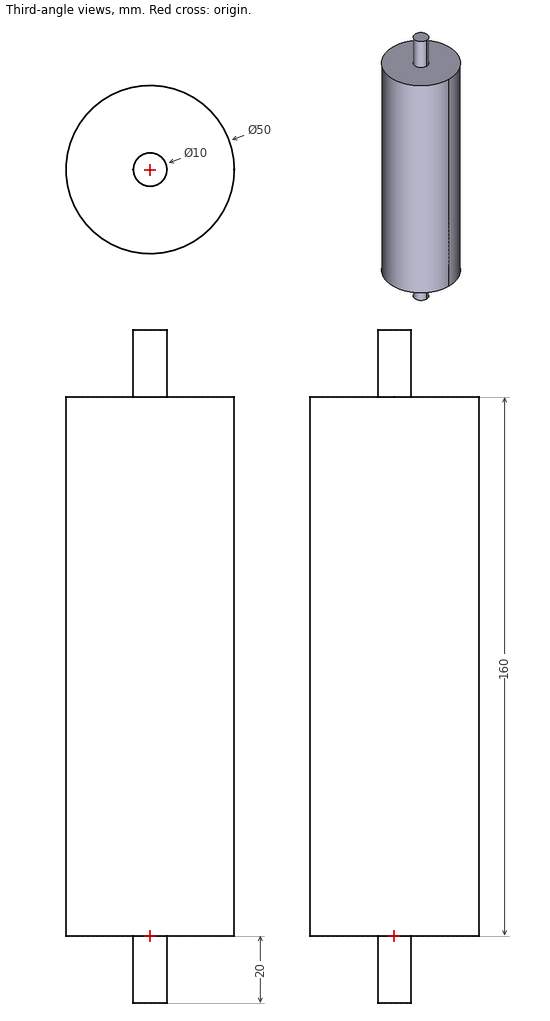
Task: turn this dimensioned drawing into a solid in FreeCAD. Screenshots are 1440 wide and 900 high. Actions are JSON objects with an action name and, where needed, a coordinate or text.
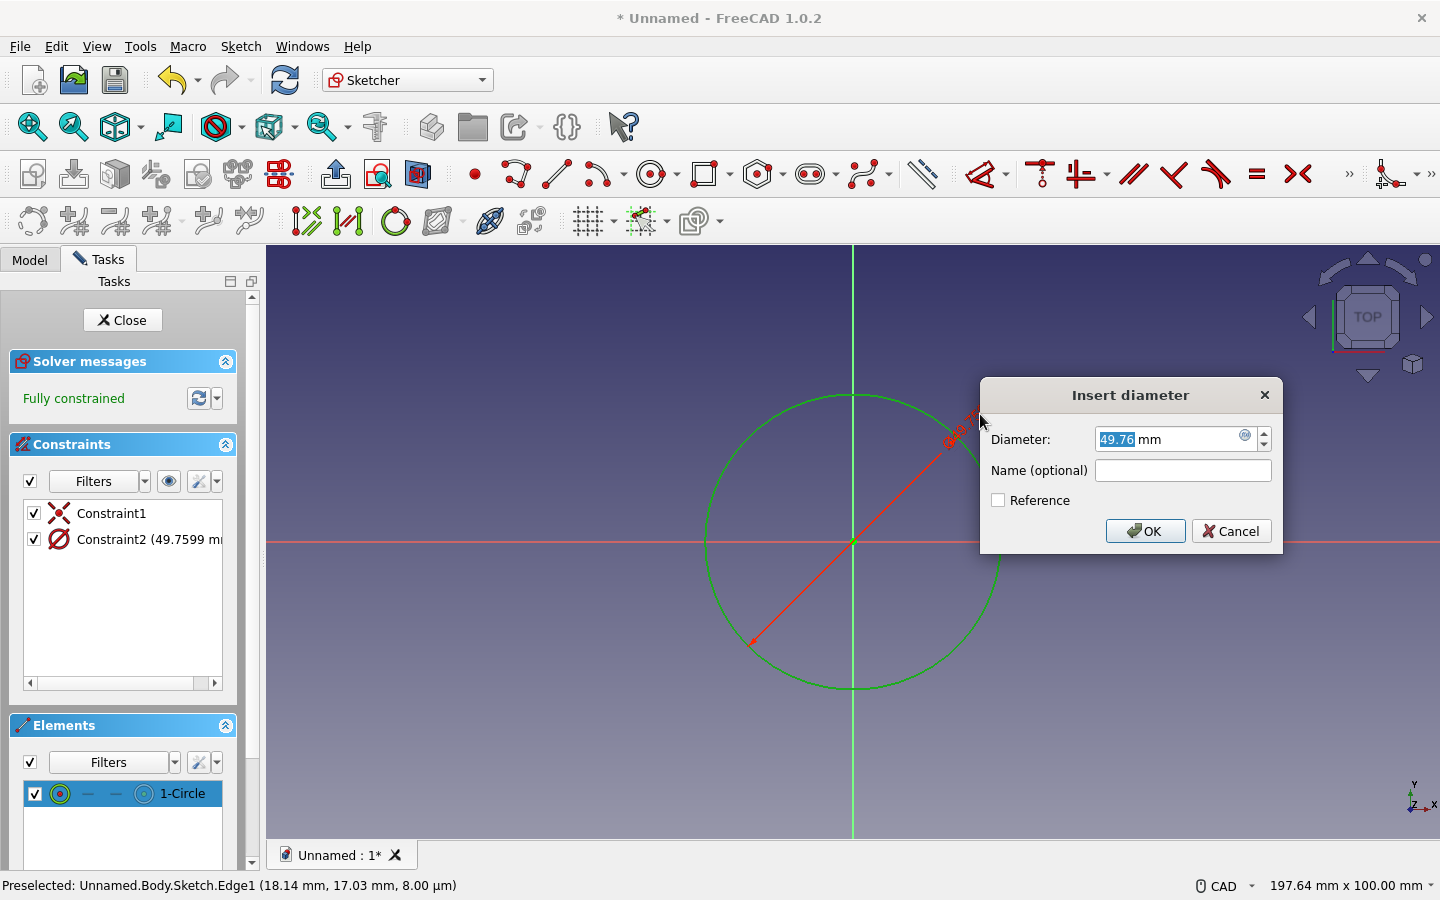
{"action": "type", "text": "50"}
{"action": "key", "text": "Return"}
{"action": "key", "text": "Escape"}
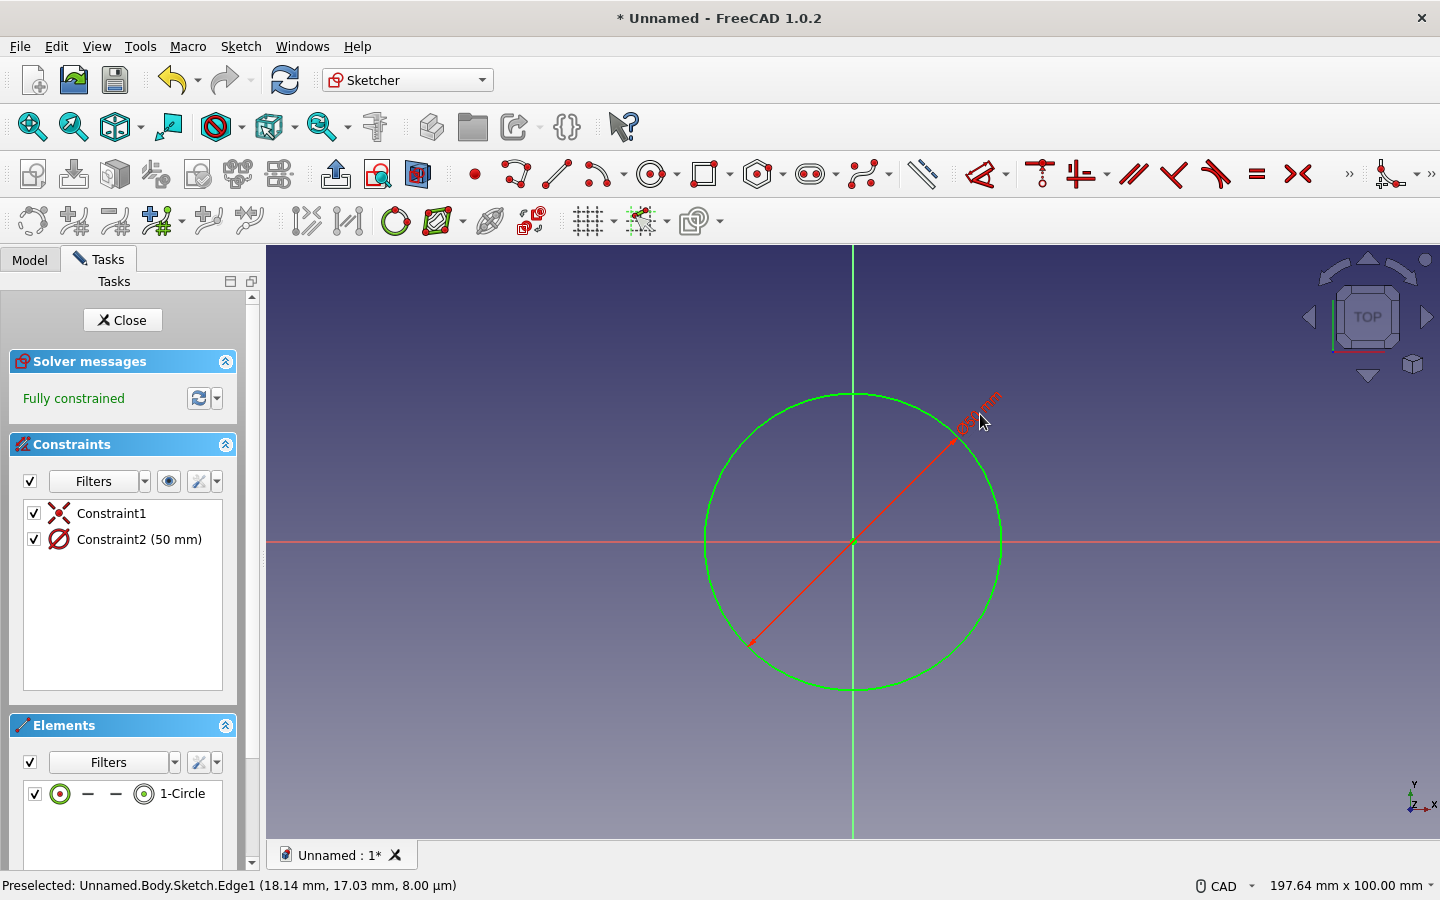
{"action": "left_click", "coordinate": [123, 320]}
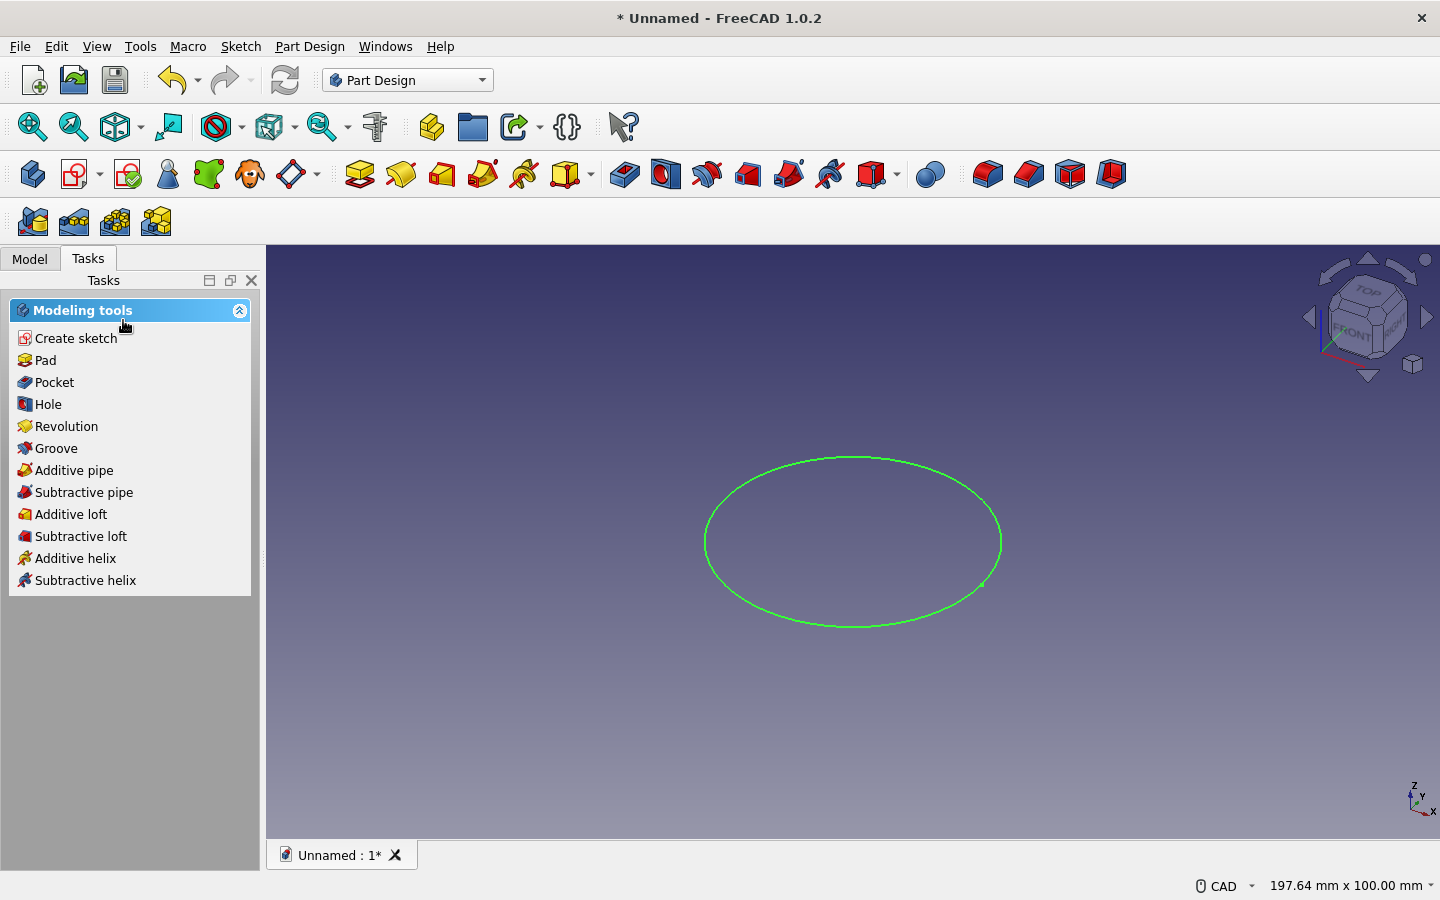
{"action": "left_click", "coordinate": [360, 174]}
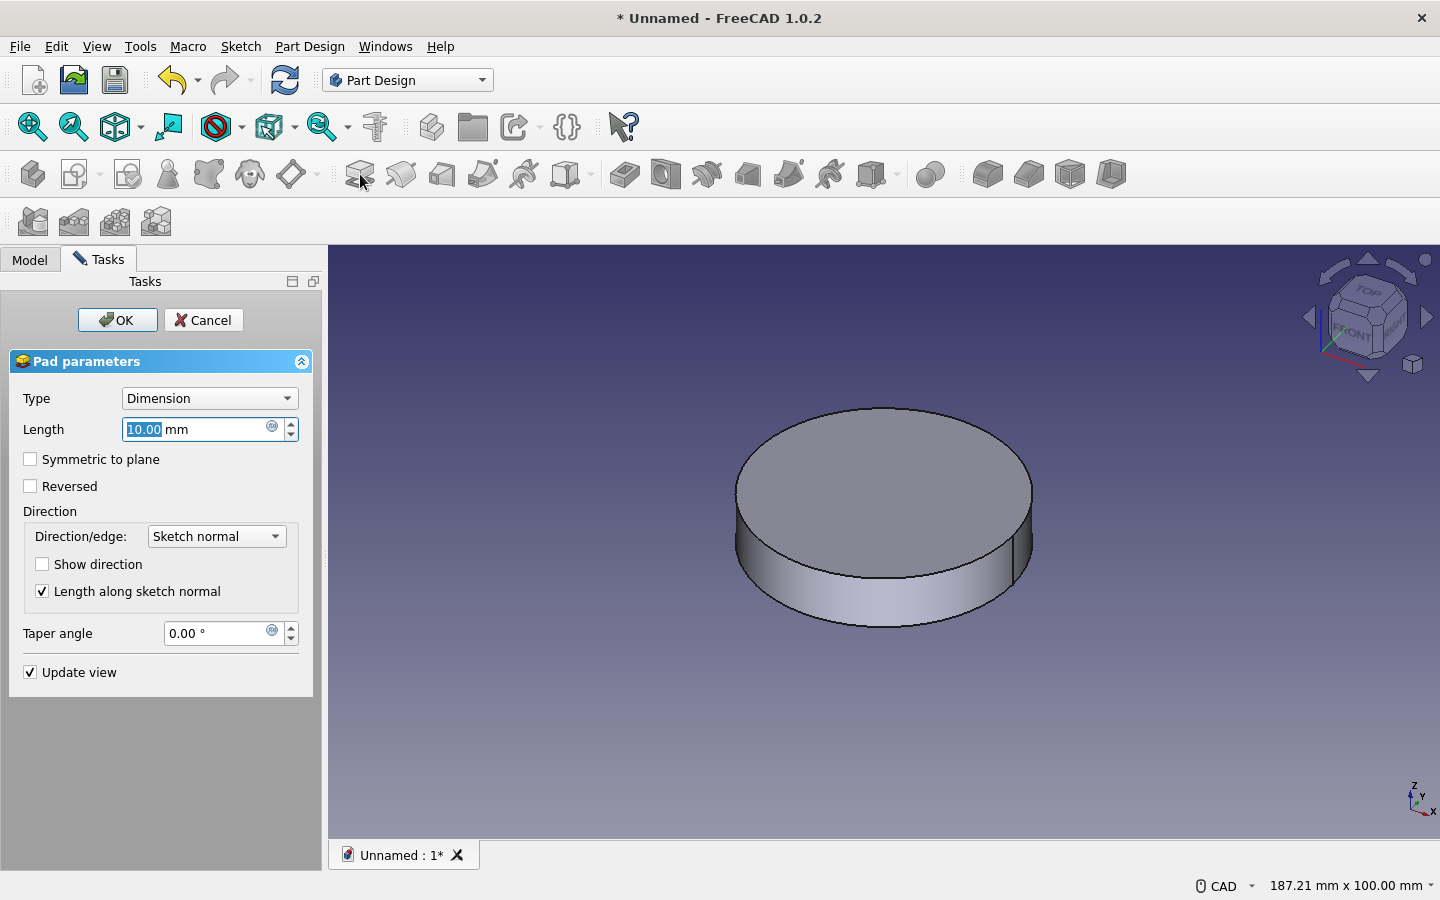
{"action": "type", "text": "160"}
{"action": "key", "text": "Tab"}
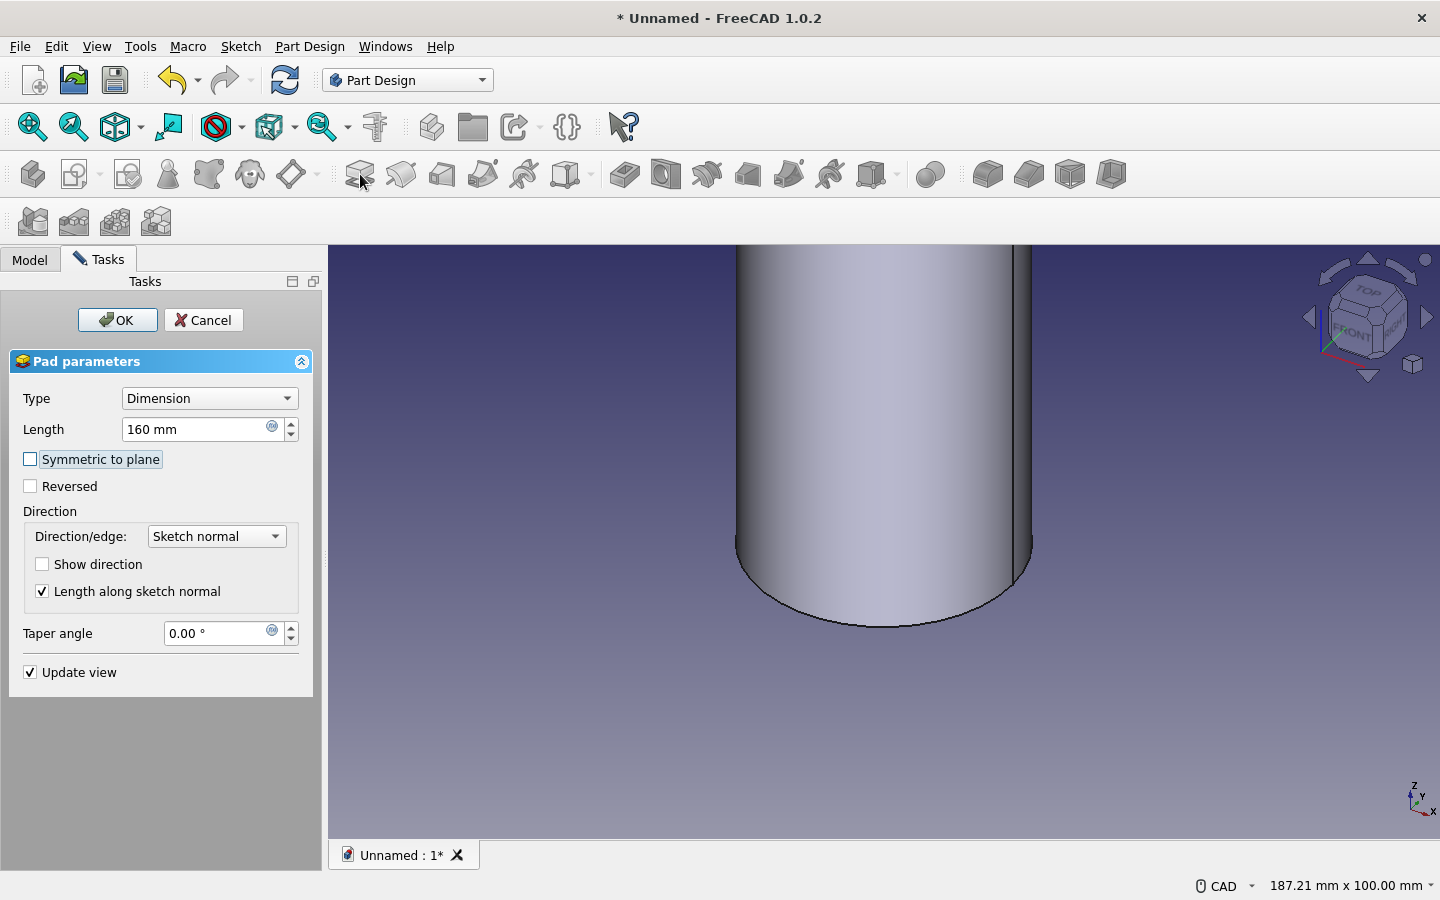
{"action": "left_click", "coordinate": [118, 320]}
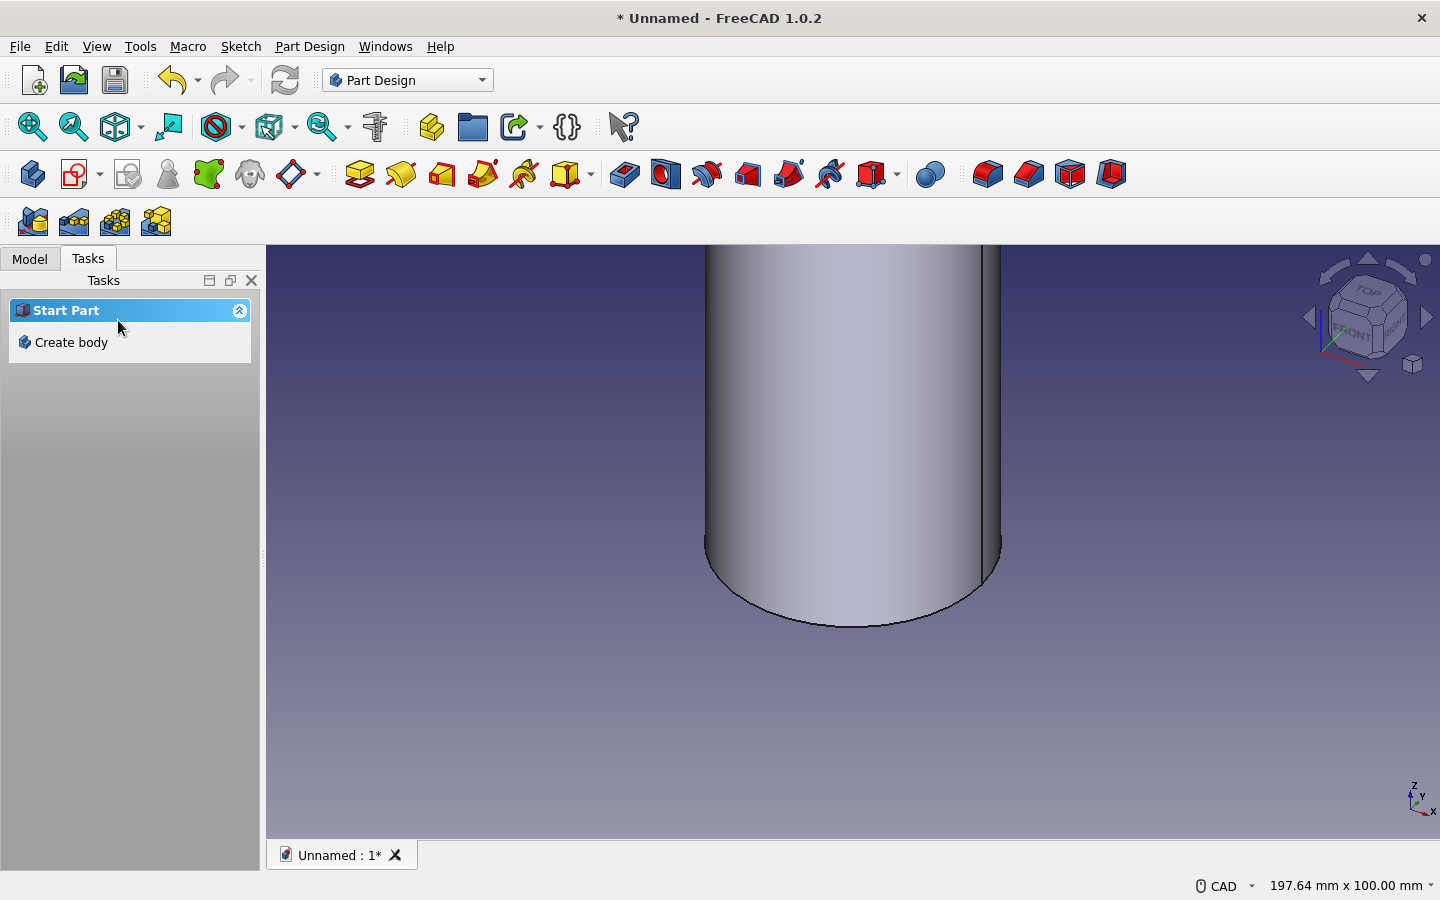
{"action": "key", "text": "v f"}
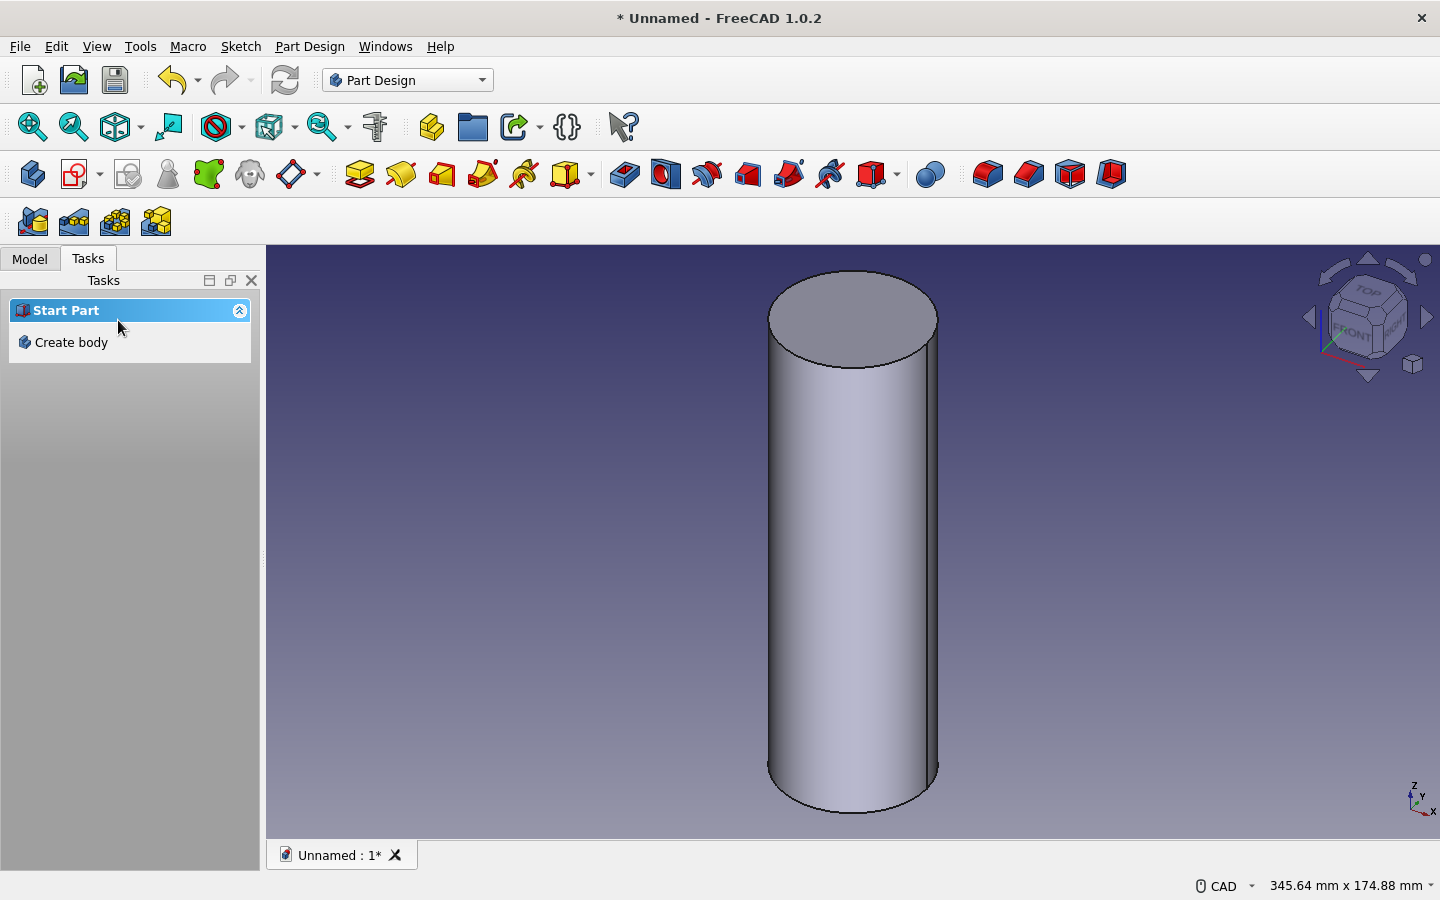
{"action": "key", "text": "5"}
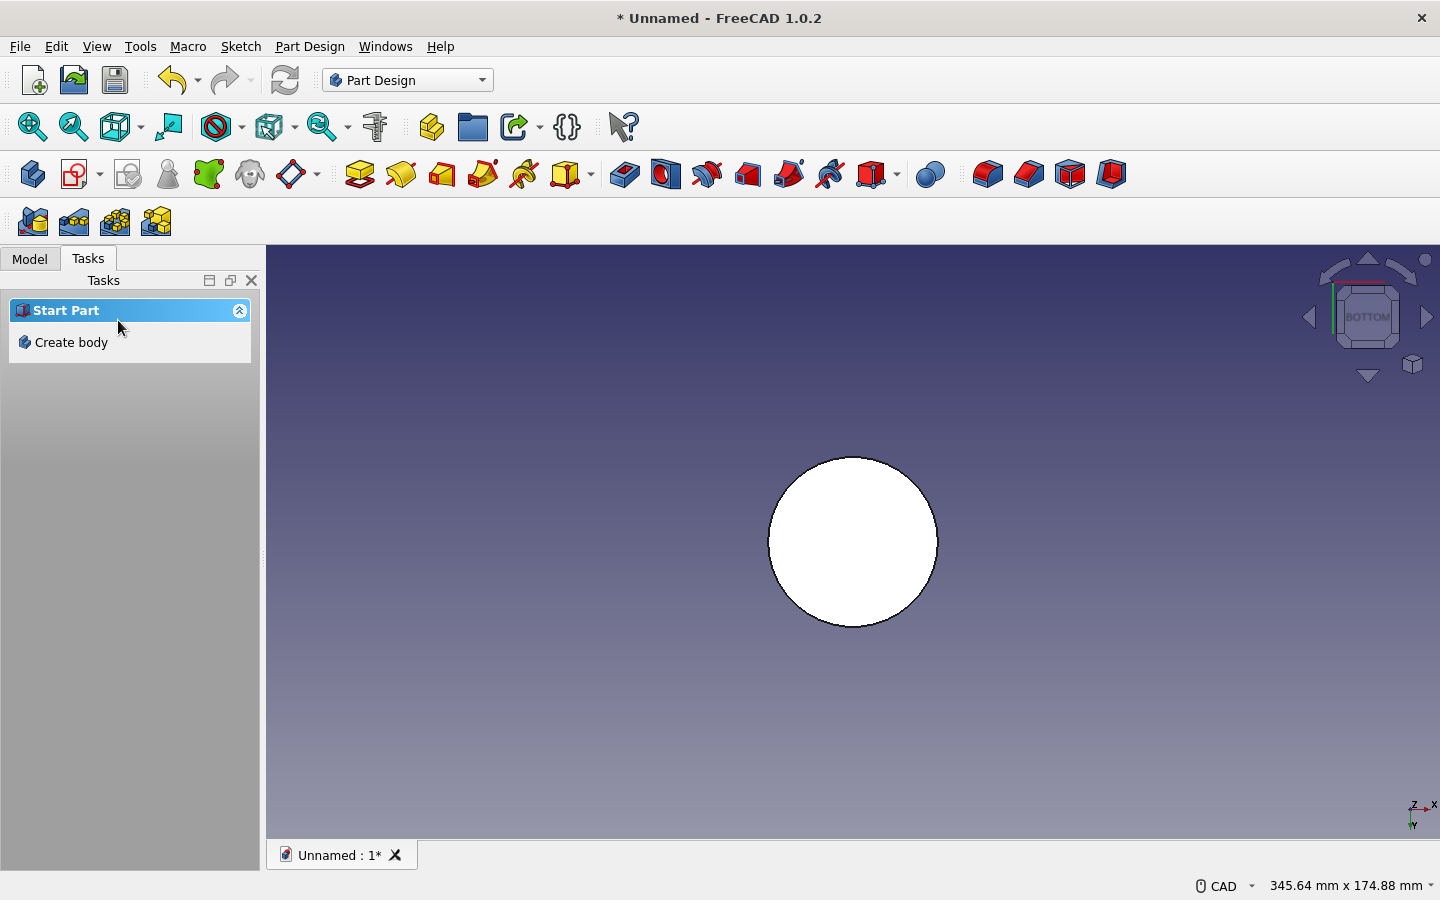
{"action": "key", "text": "v f"}